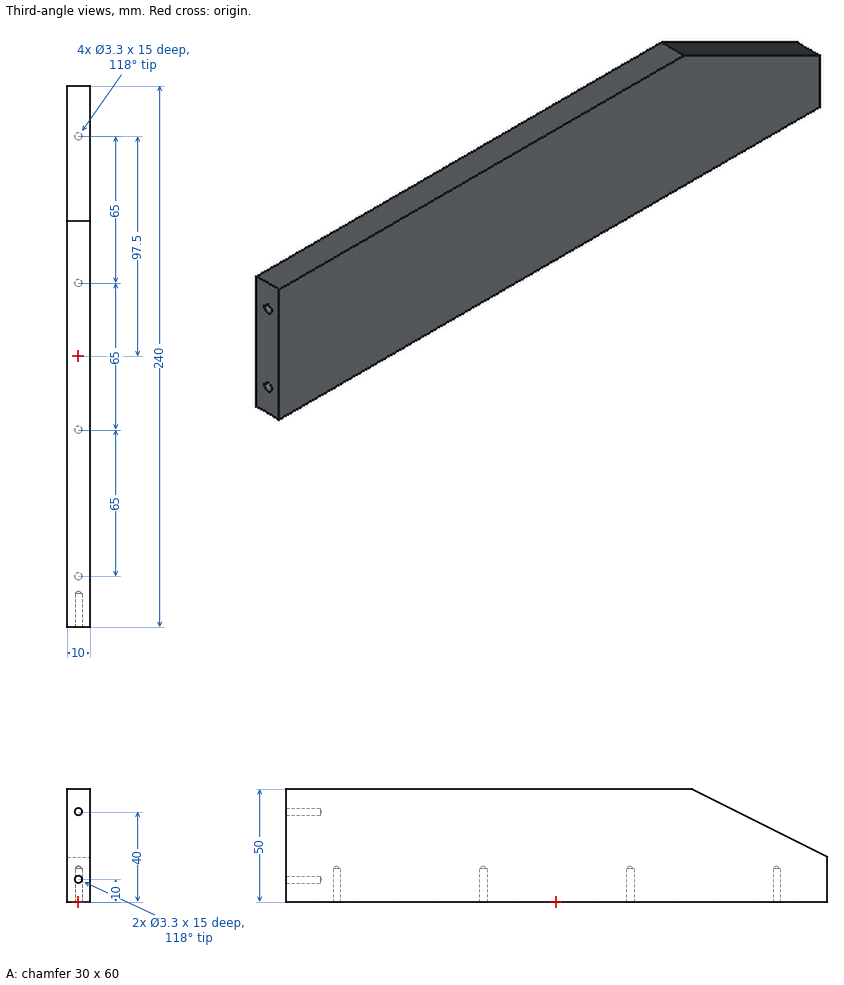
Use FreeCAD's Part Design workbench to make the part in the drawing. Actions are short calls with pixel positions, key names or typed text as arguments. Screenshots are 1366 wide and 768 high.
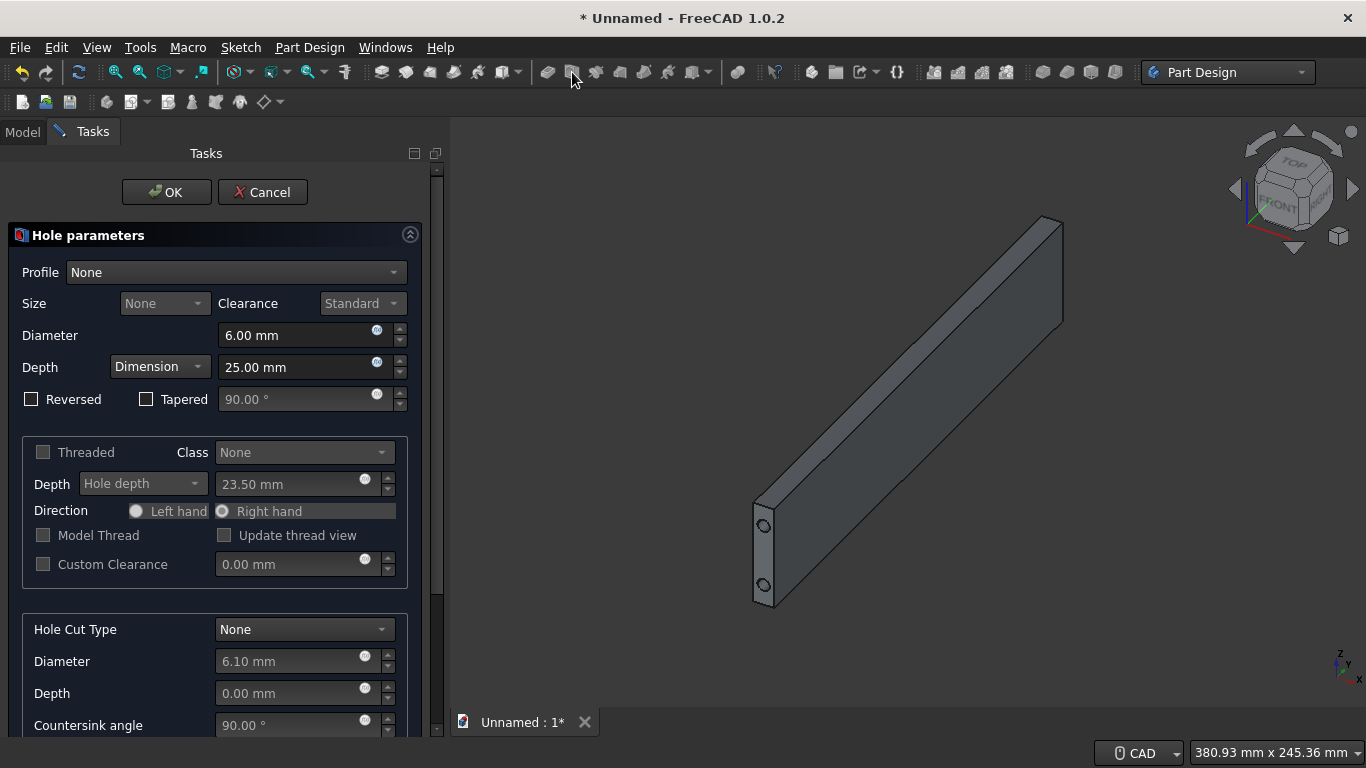
triple_click(305, 335)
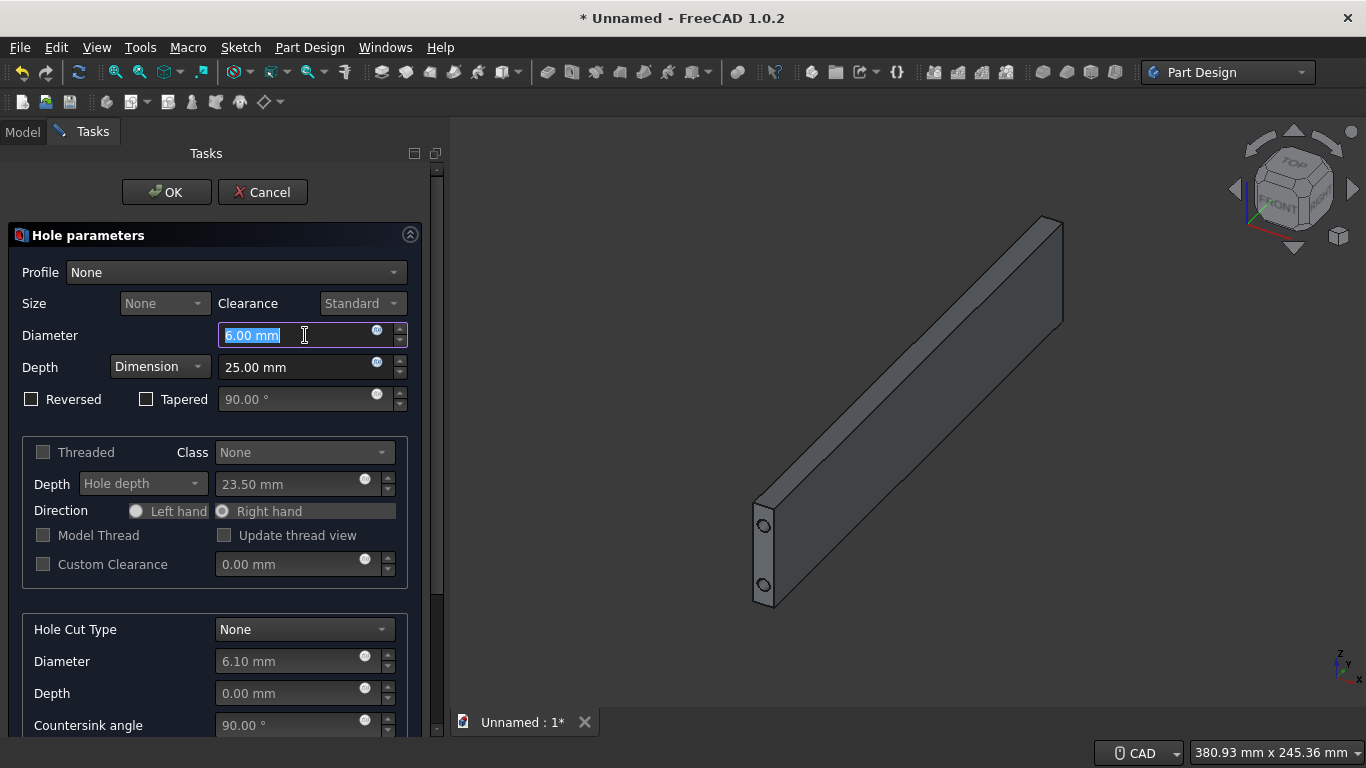
text(3.3)
key(Tab)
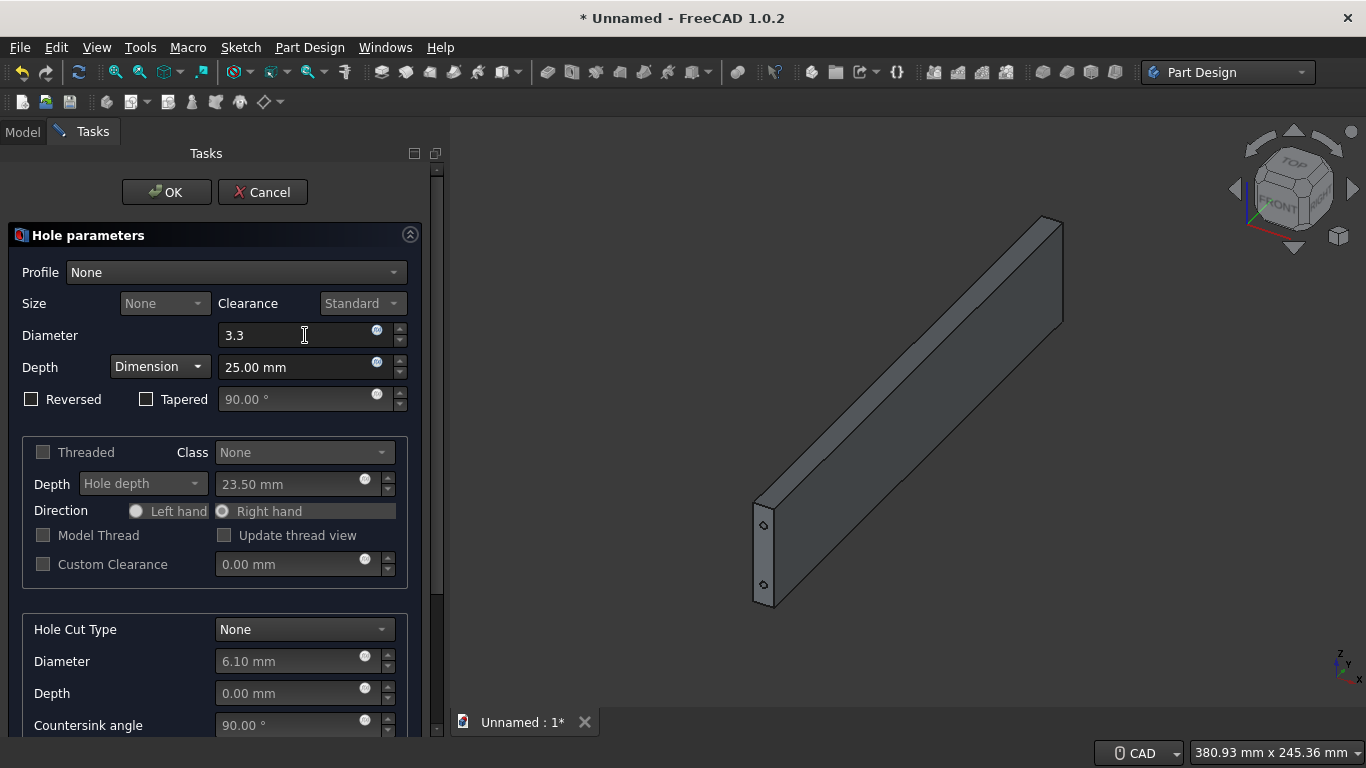
triple_click(305, 367)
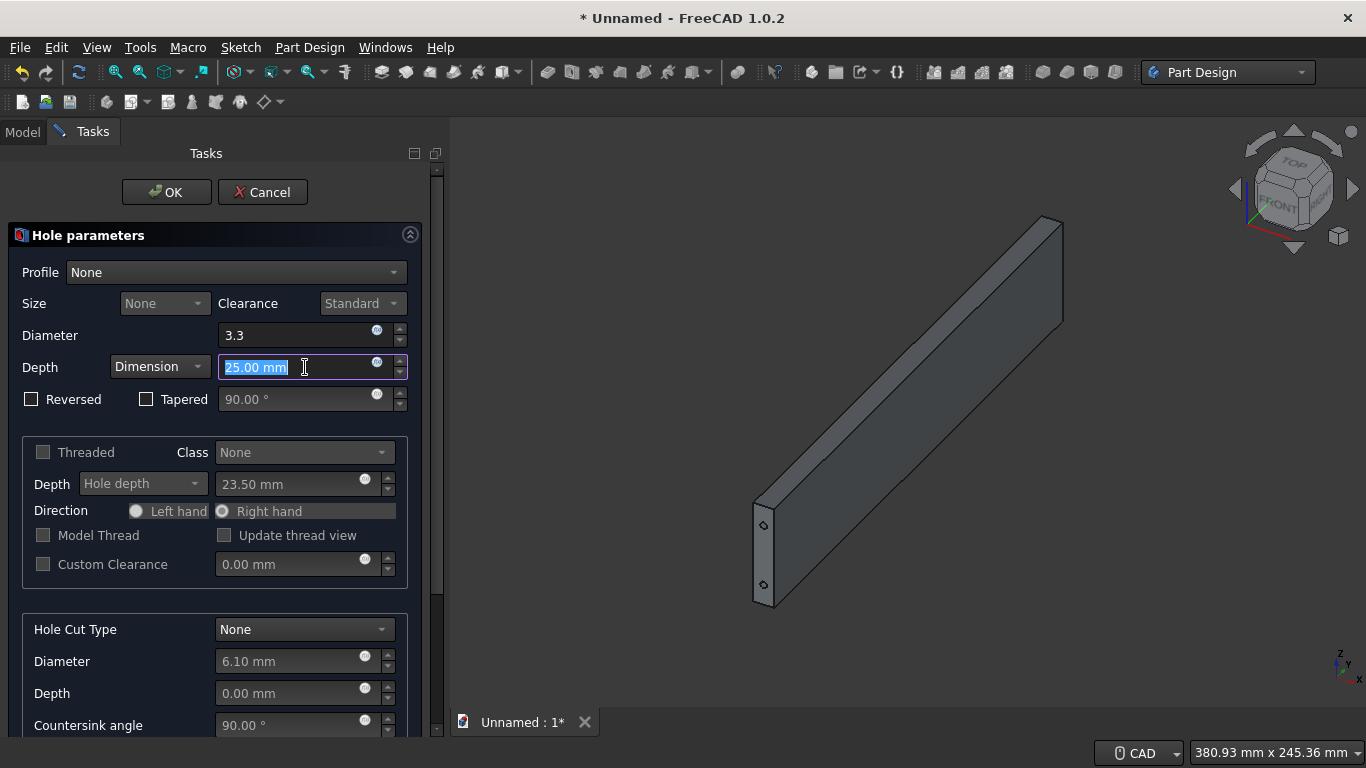
text(15)
key(Tab)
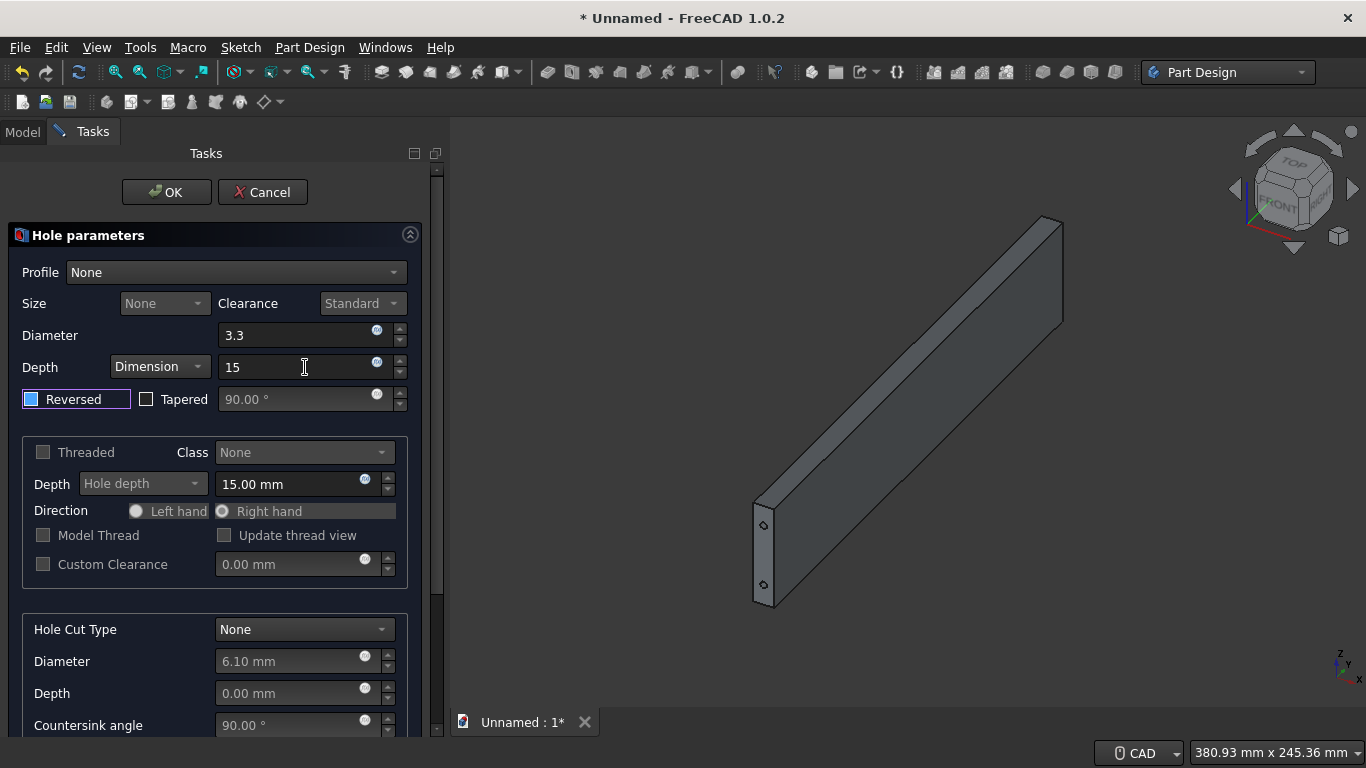
click(167, 192)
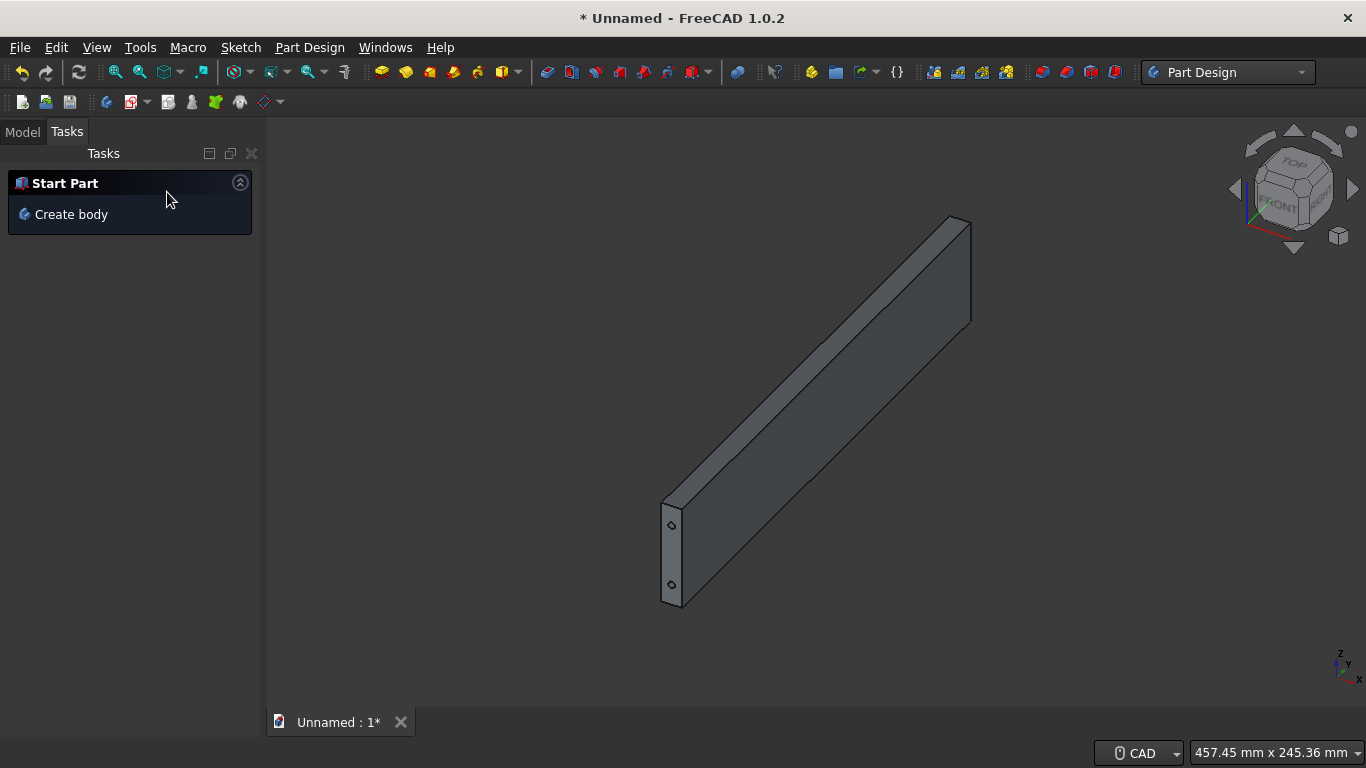
key(0)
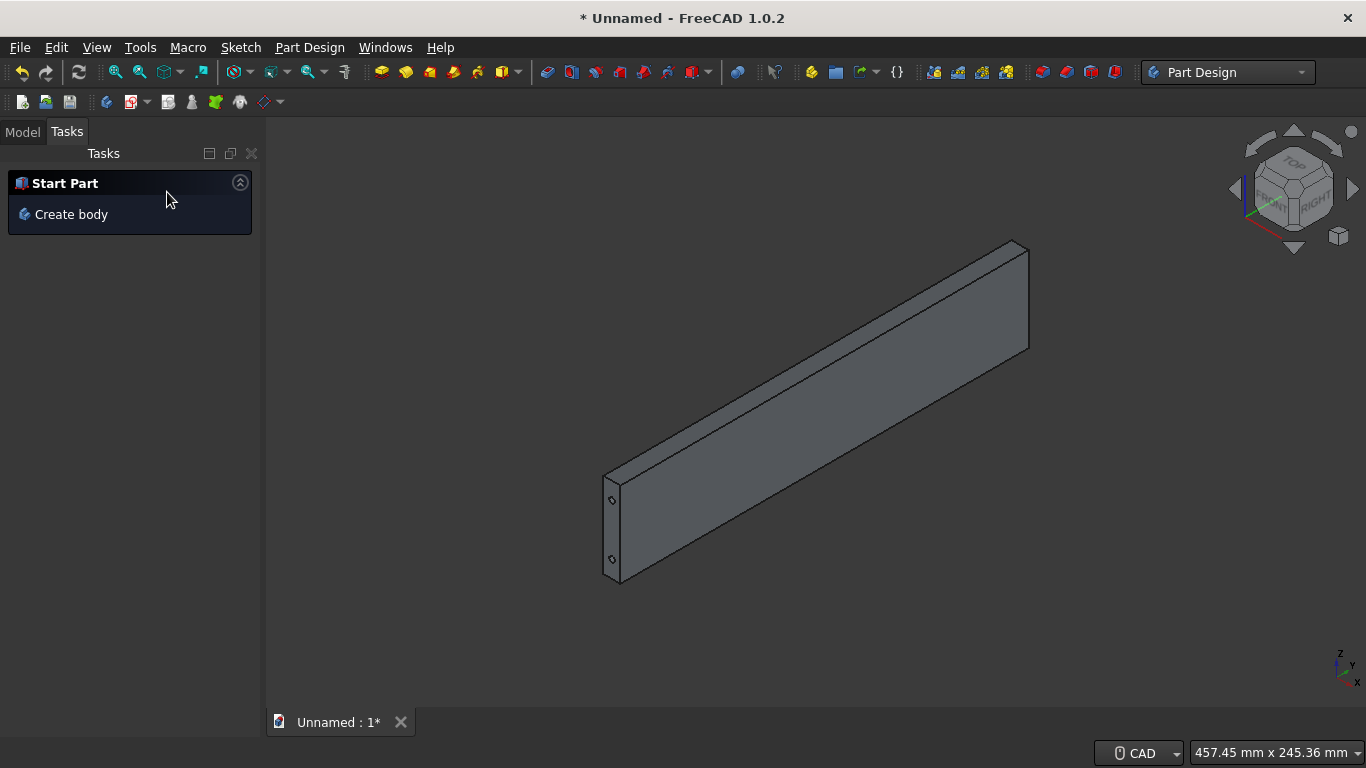
key(2)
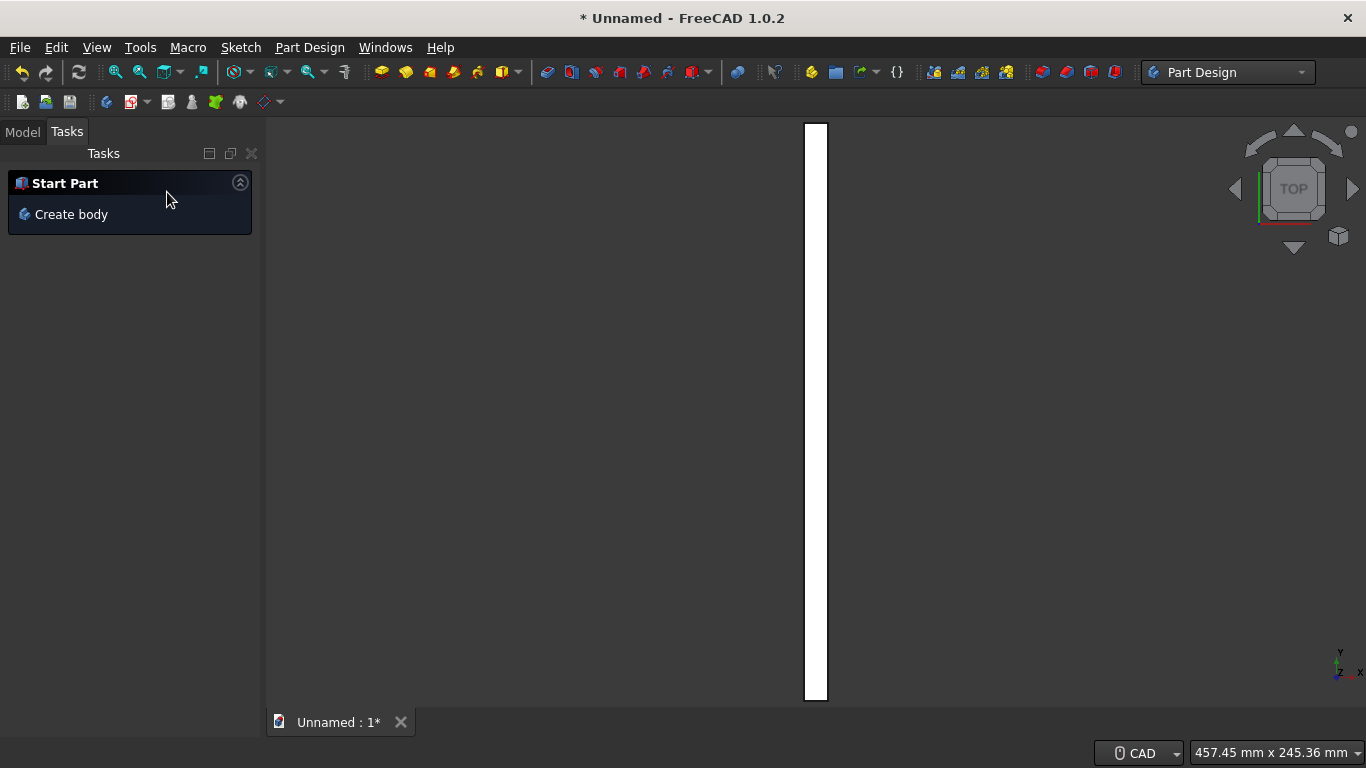
key(1)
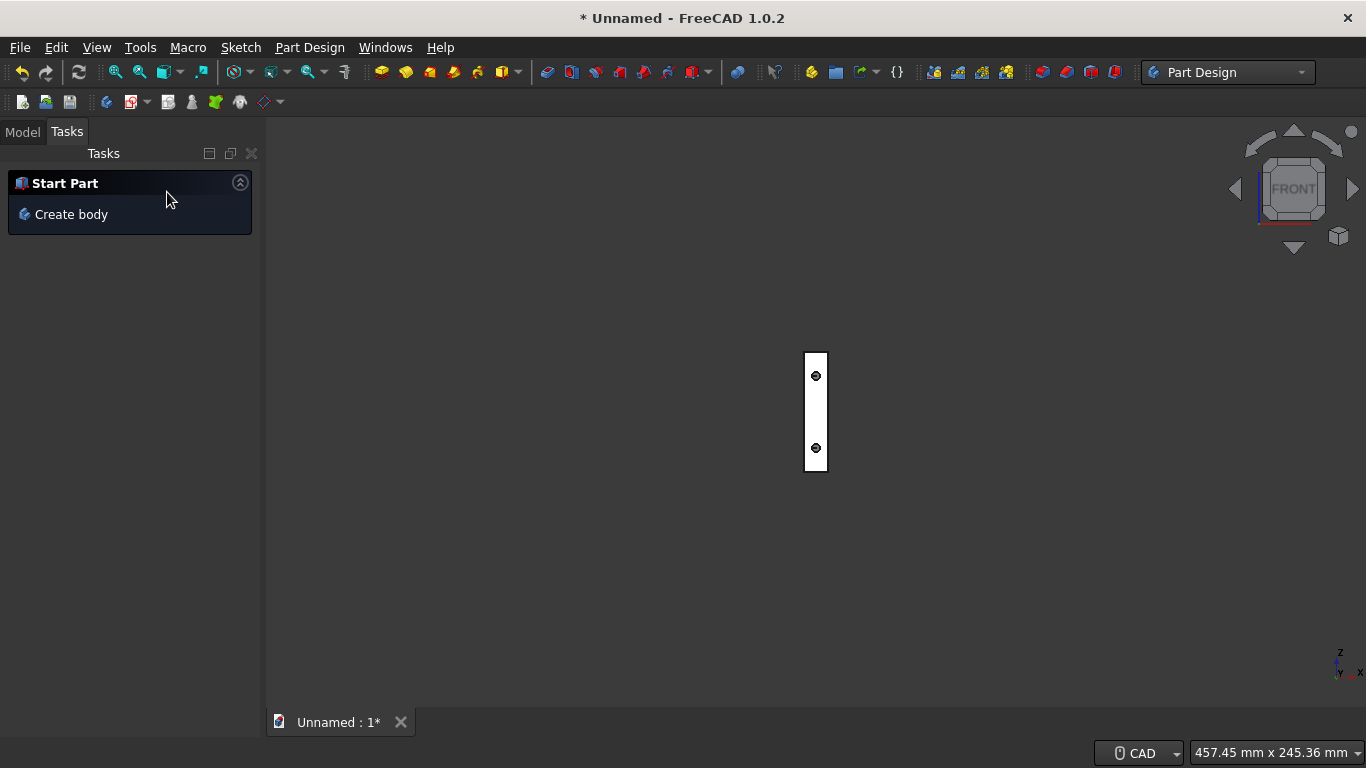
key(v)
key(f)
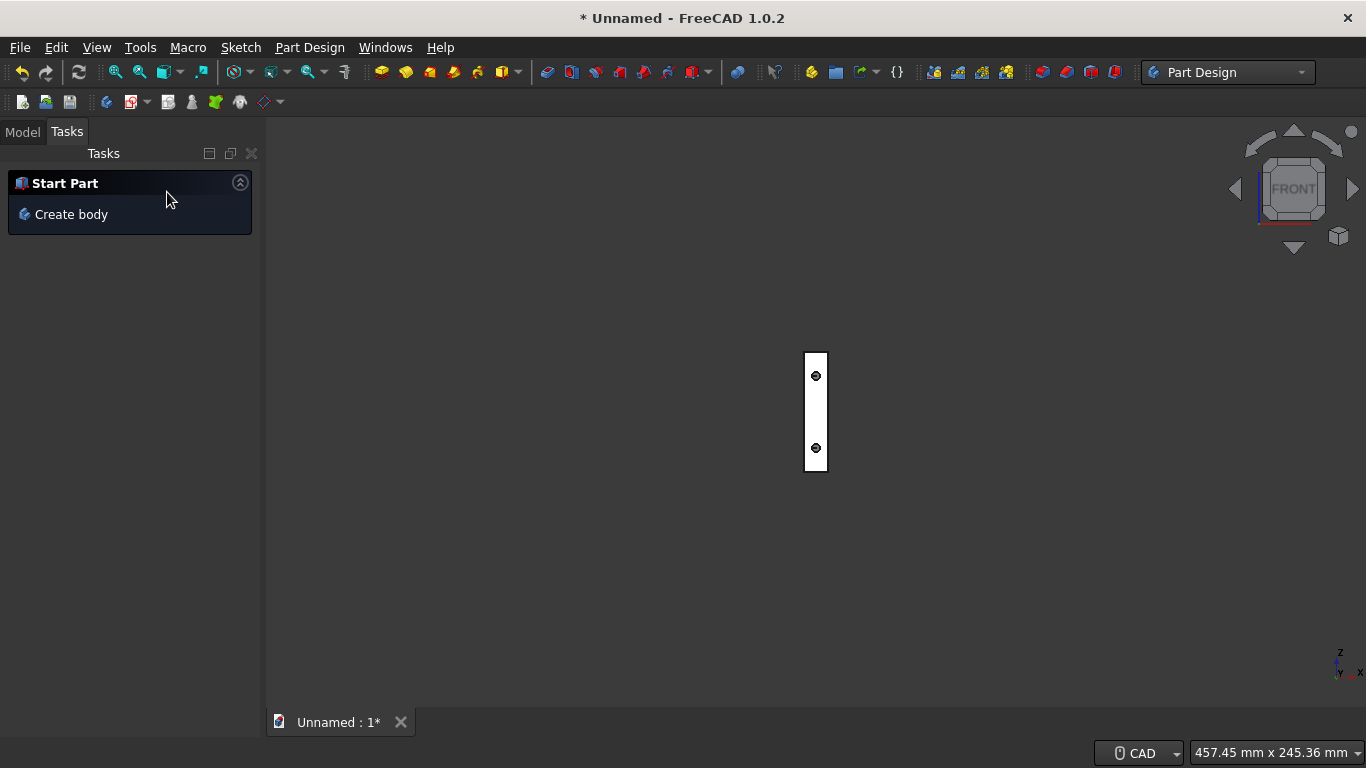
key(3)